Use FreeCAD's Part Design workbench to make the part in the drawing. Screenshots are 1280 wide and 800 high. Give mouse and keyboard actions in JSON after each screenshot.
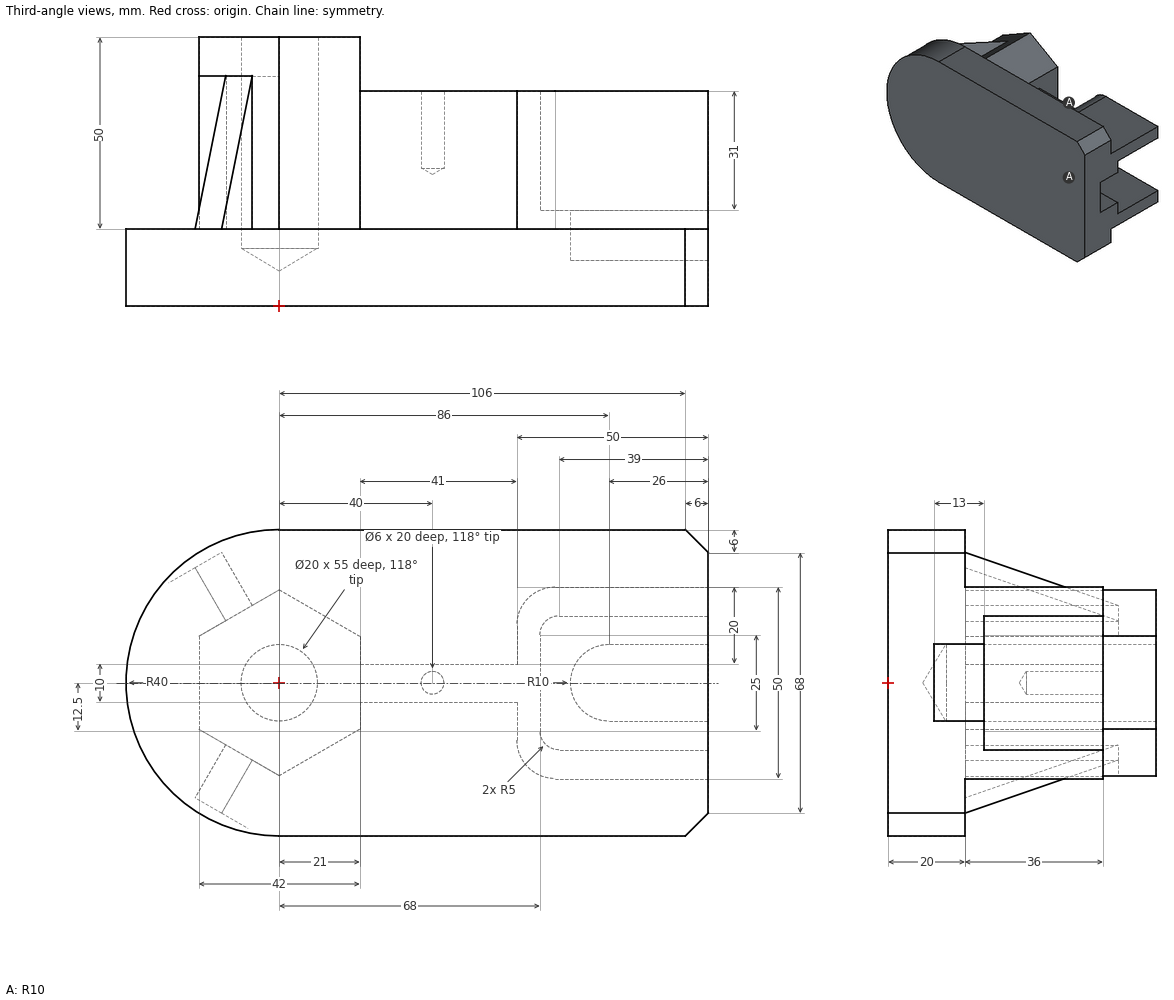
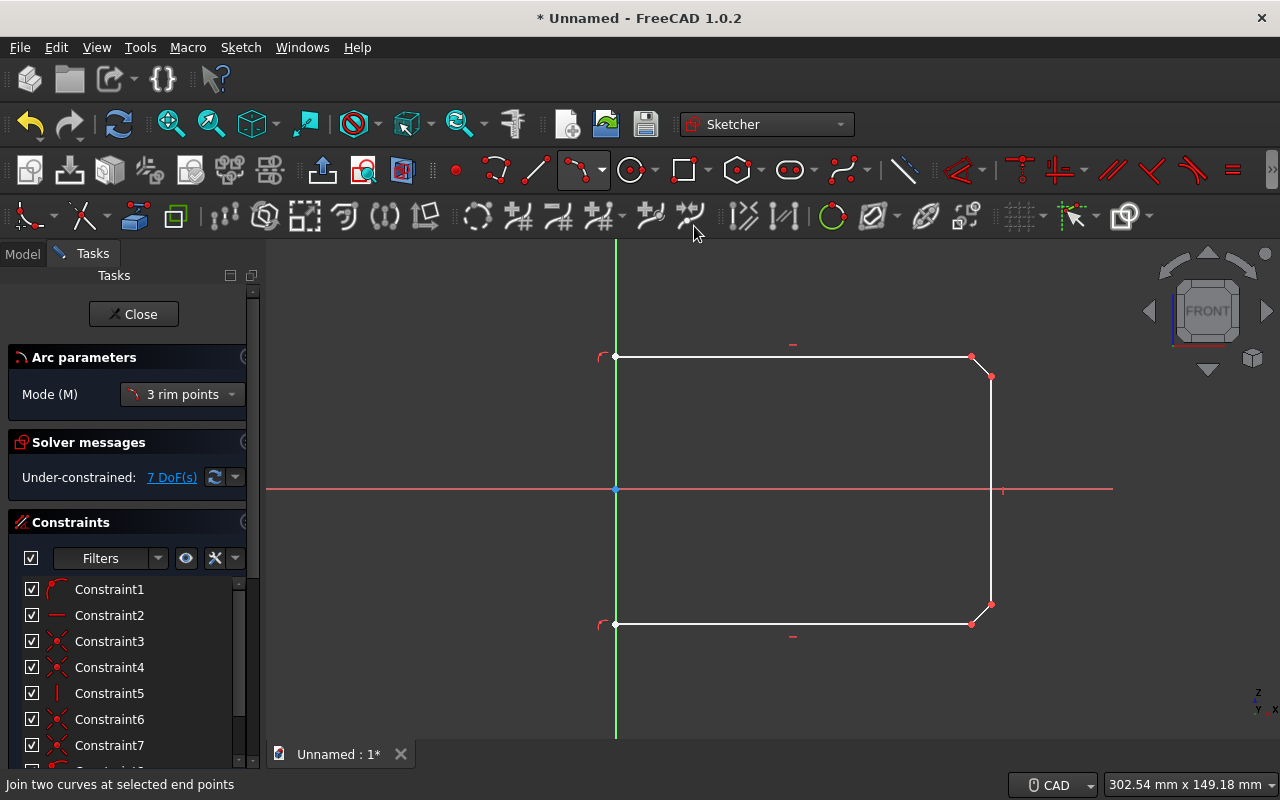
{"action": "left_click", "coordinate": [616, 624]}
{"action": "left_click", "coordinate": [616, 357]}
{"action": "left_click", "coordinate": [488, 448]}
{"action": "key", "text": "Escape"}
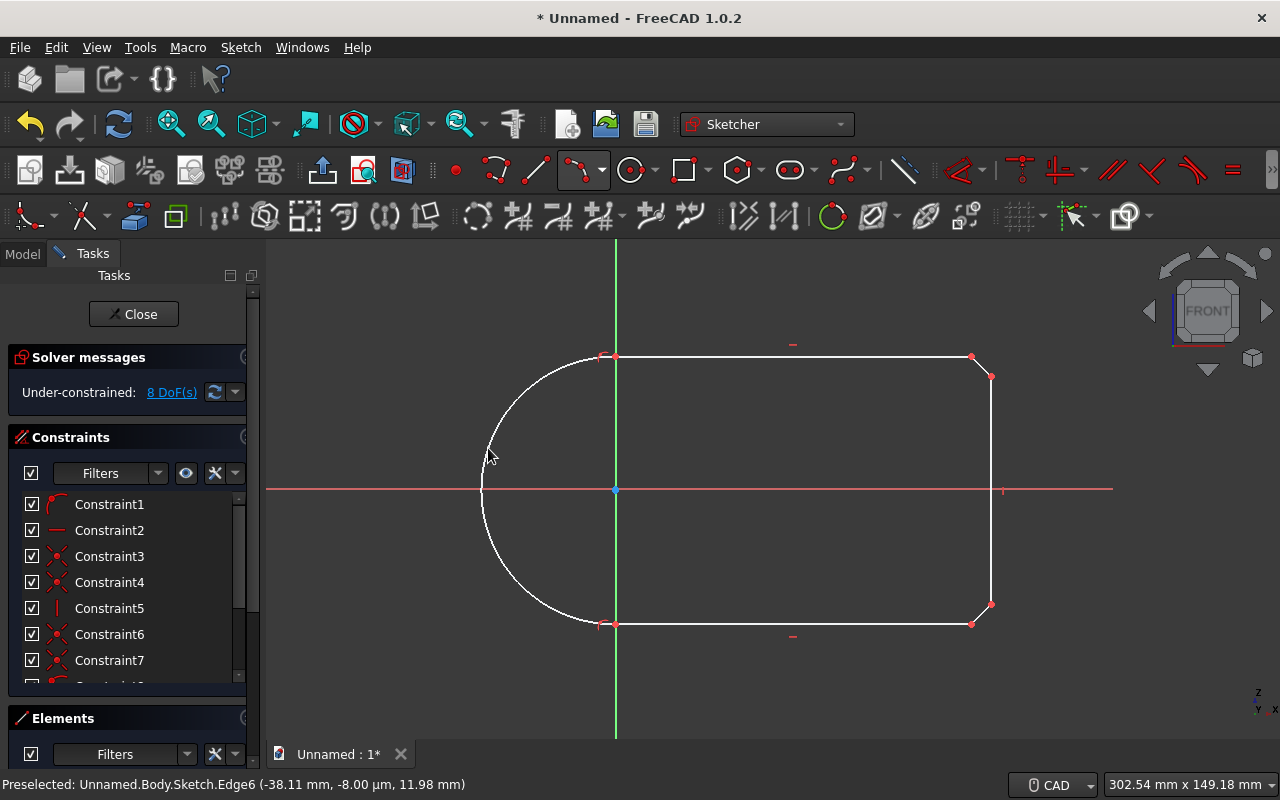
{"action": "left_click_drag", "start_coordinate": [605, 479], "coordinate": [626, 500]}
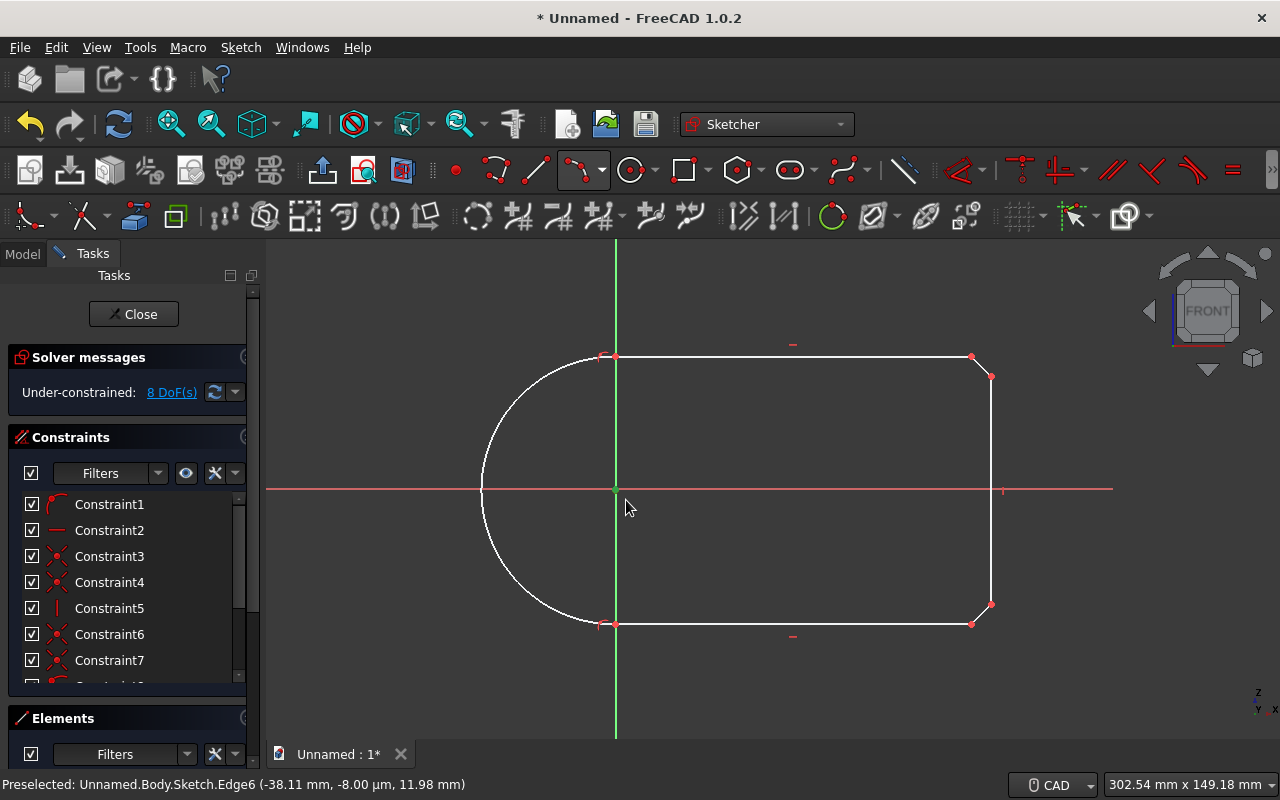
{"action": "left_click", "coordinate": [1020, 170]}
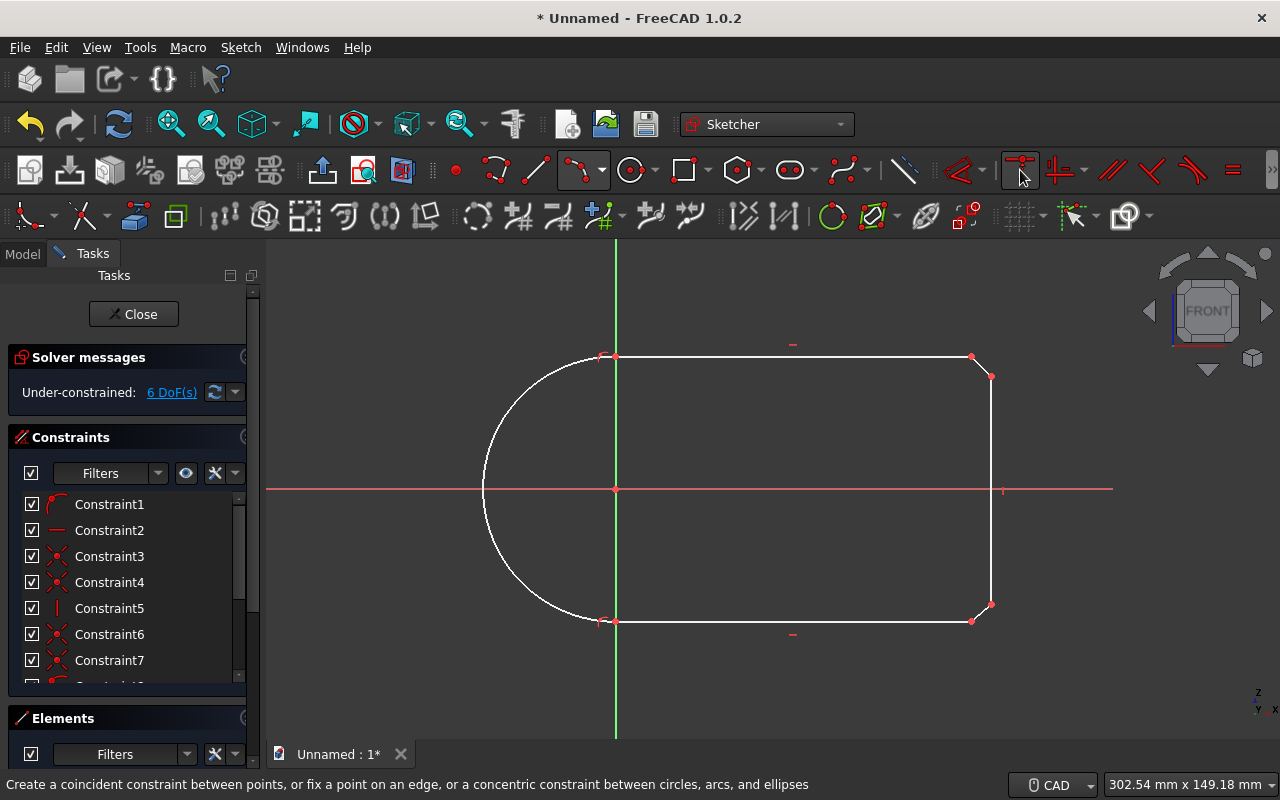
{"action": "left_click", "coordinate": [958, 170]}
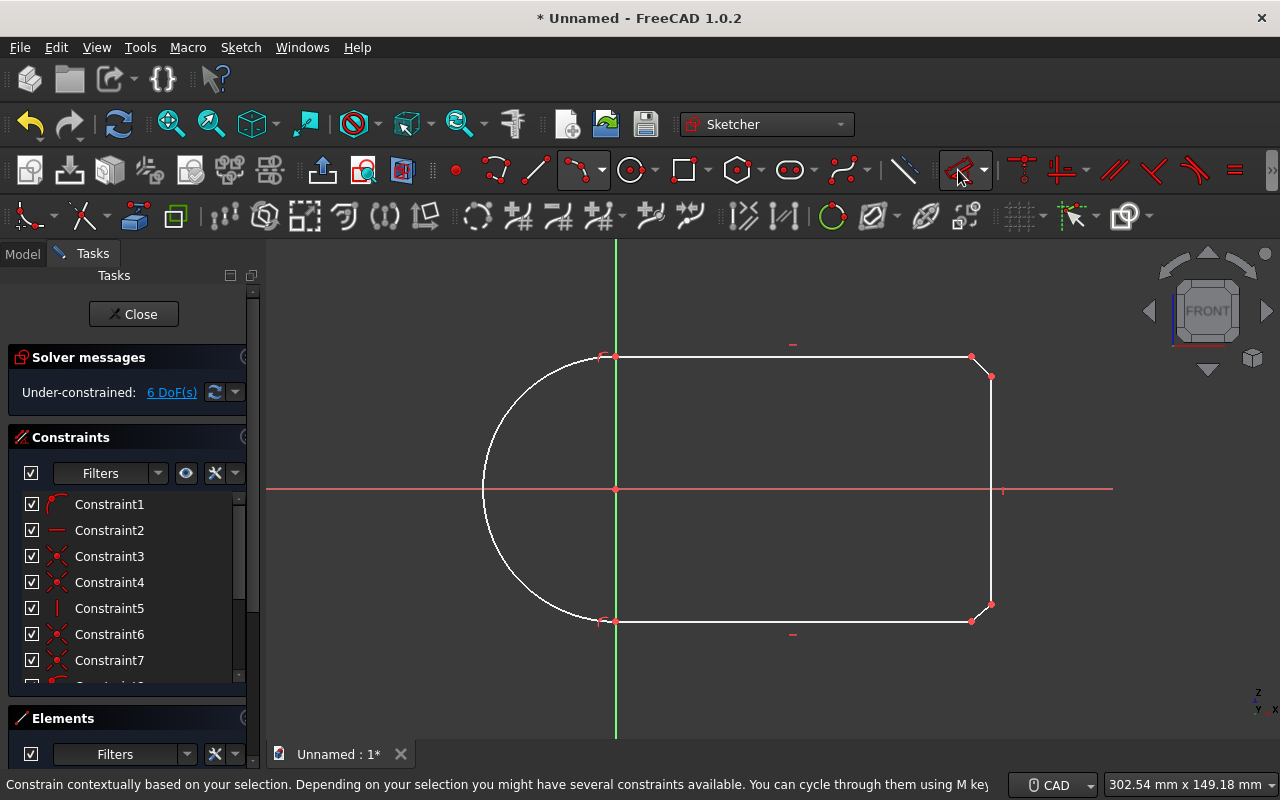
{"action": "left_click", "coordinate": [508, 411]}
{"action": "left_click", "coordinate": [482, 392]}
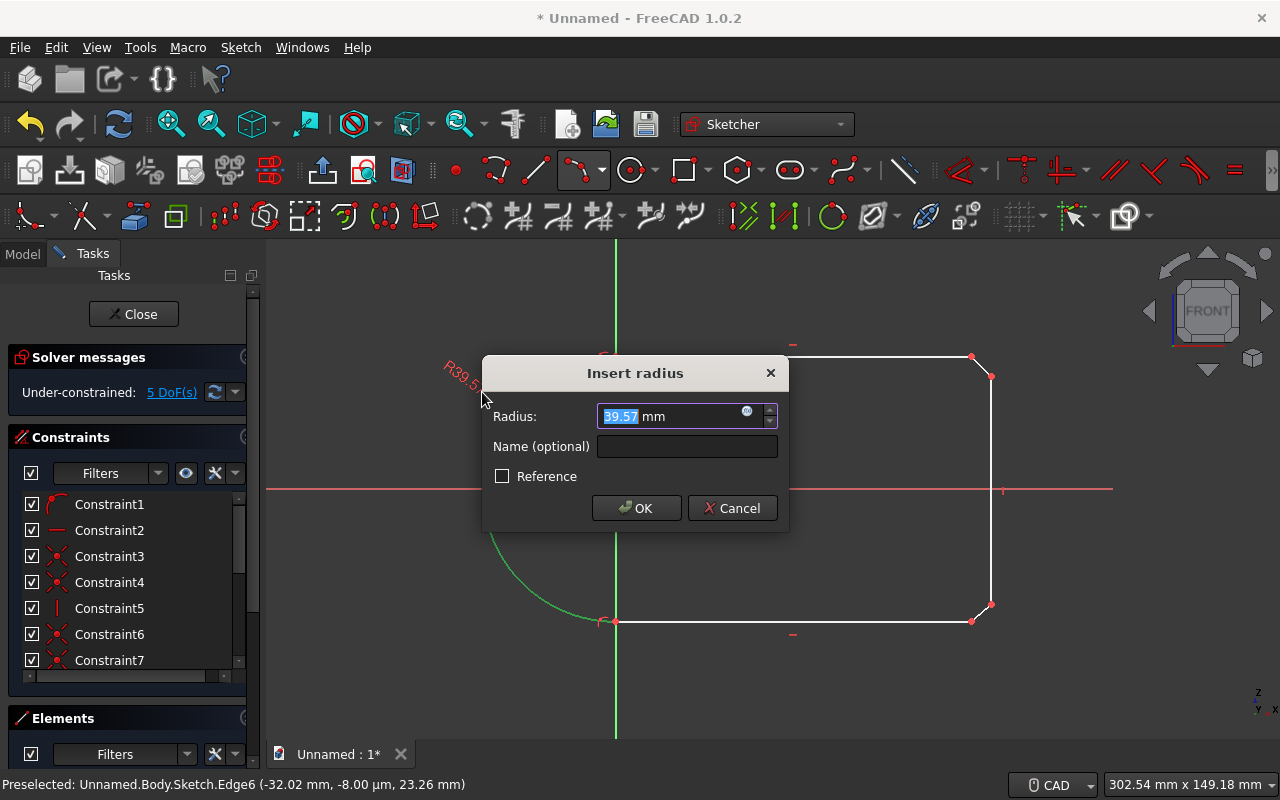
{"action": "type", "text": "40"}
{"action": "key", "text": "Return"}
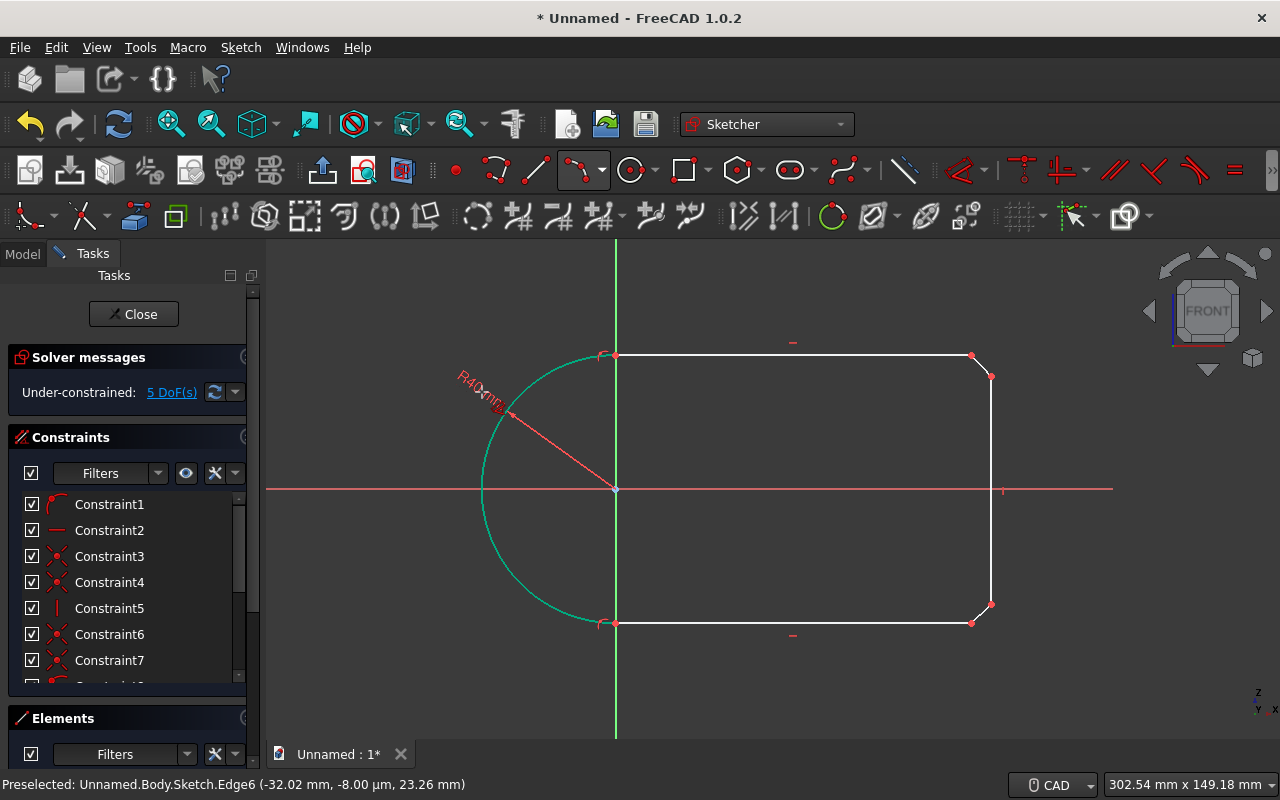
{"action": "left_click", "coordinate": [991, 445]}
{"action": "left_click", "coordinate": [1025, 438]}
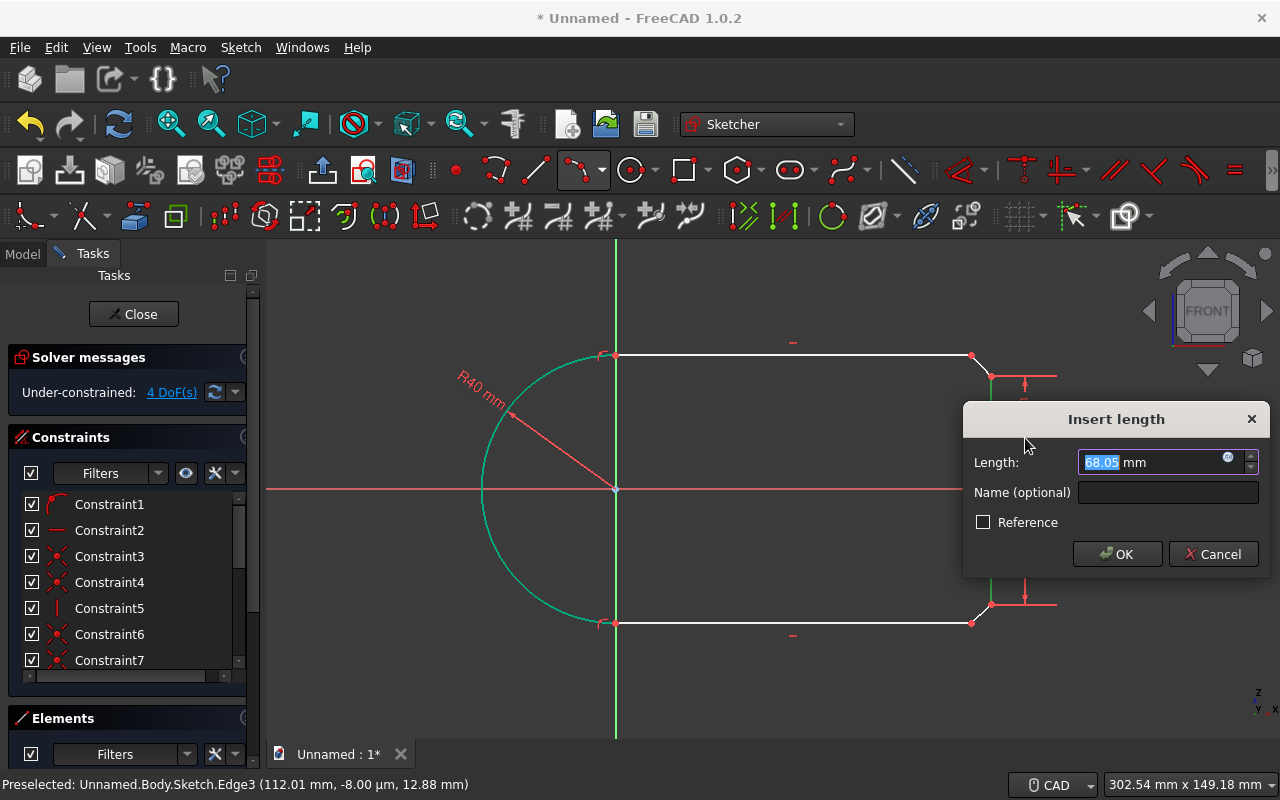
{"action": "type", "text": "68"}
{"action": "key", "text": "Return"}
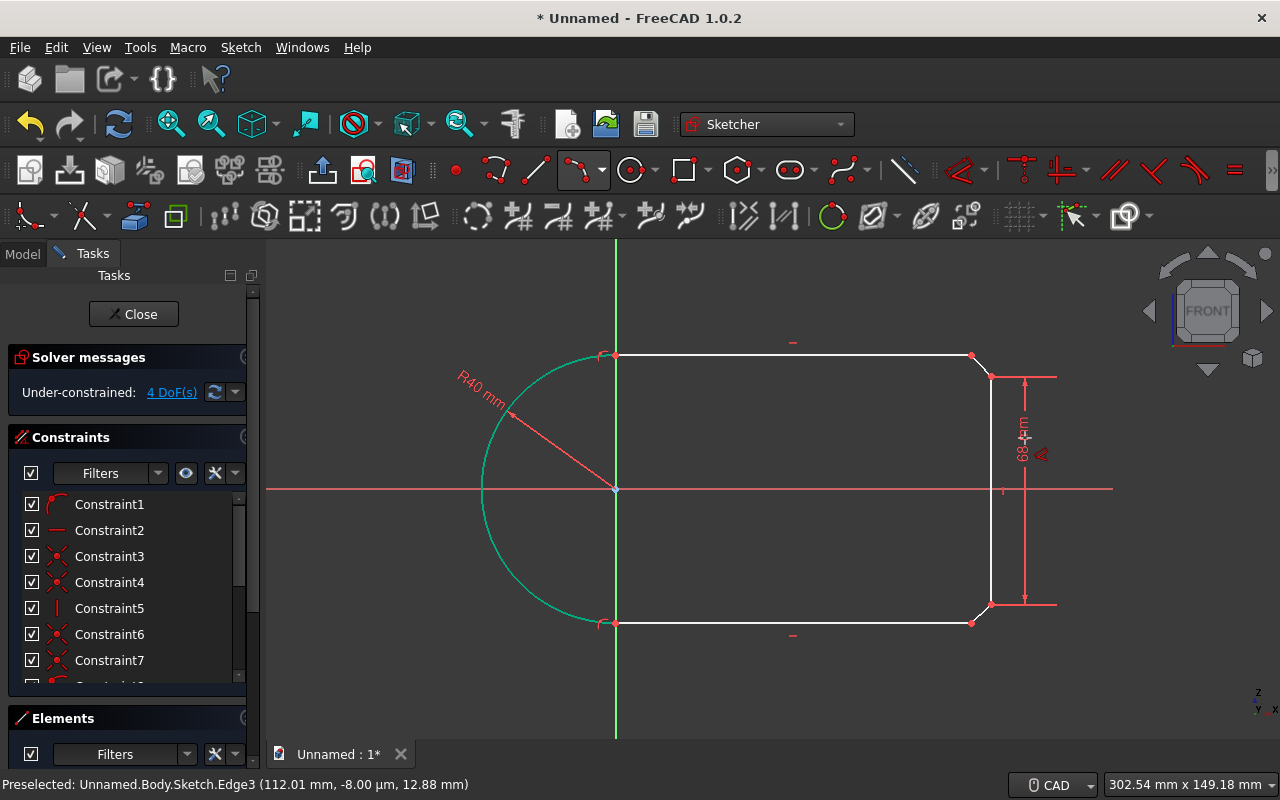
{"action": "scroll", "coordinate": [979, 364], "scroll_direction": "up", "scroll_amount": 4}